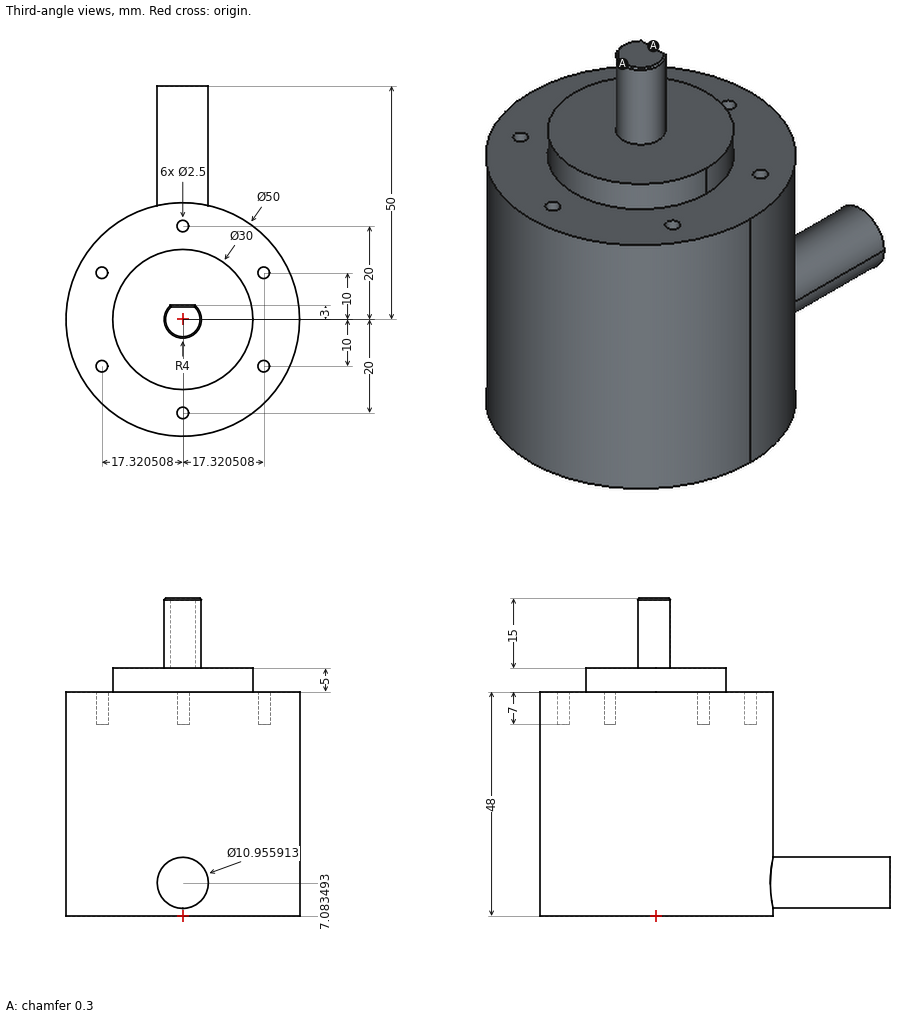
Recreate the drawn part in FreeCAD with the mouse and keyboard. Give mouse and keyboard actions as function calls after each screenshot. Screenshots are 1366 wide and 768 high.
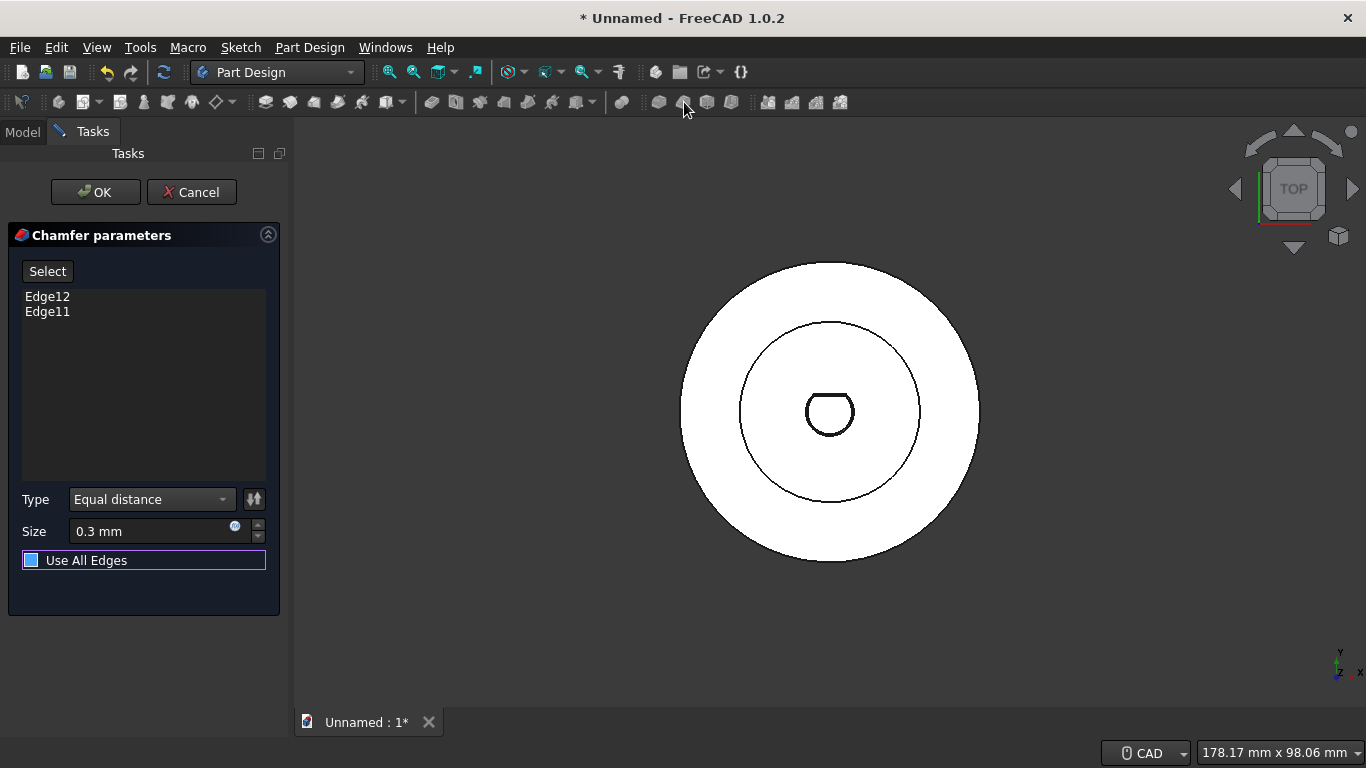
click(96, 192)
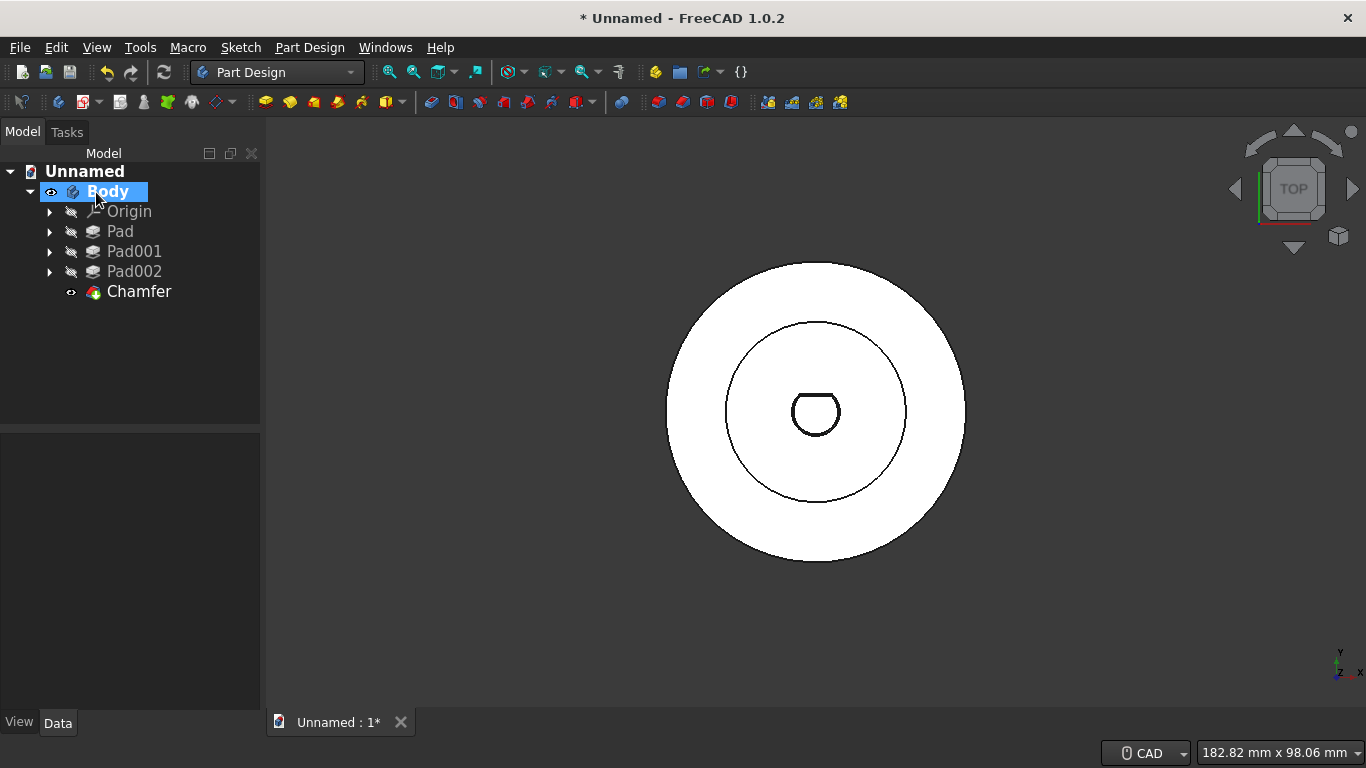
click(84, 102)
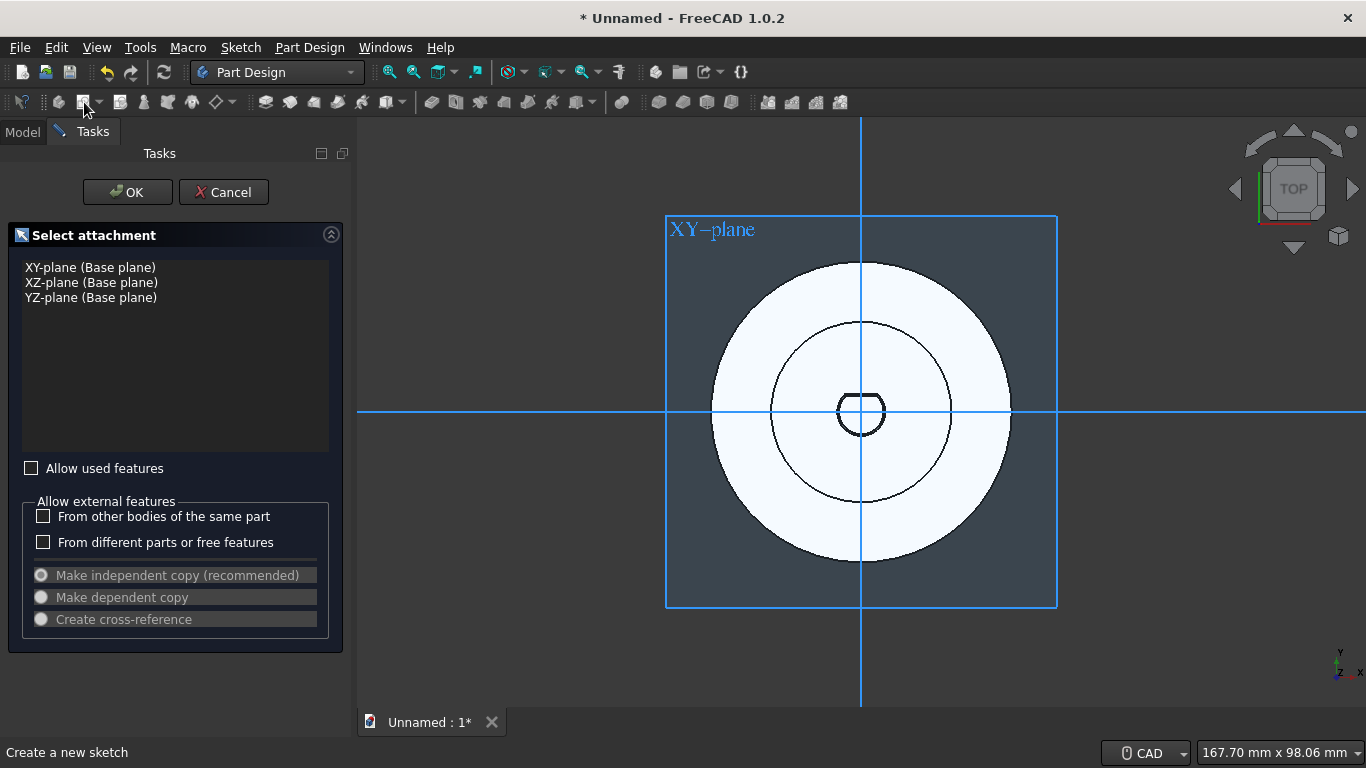
click(82, 282)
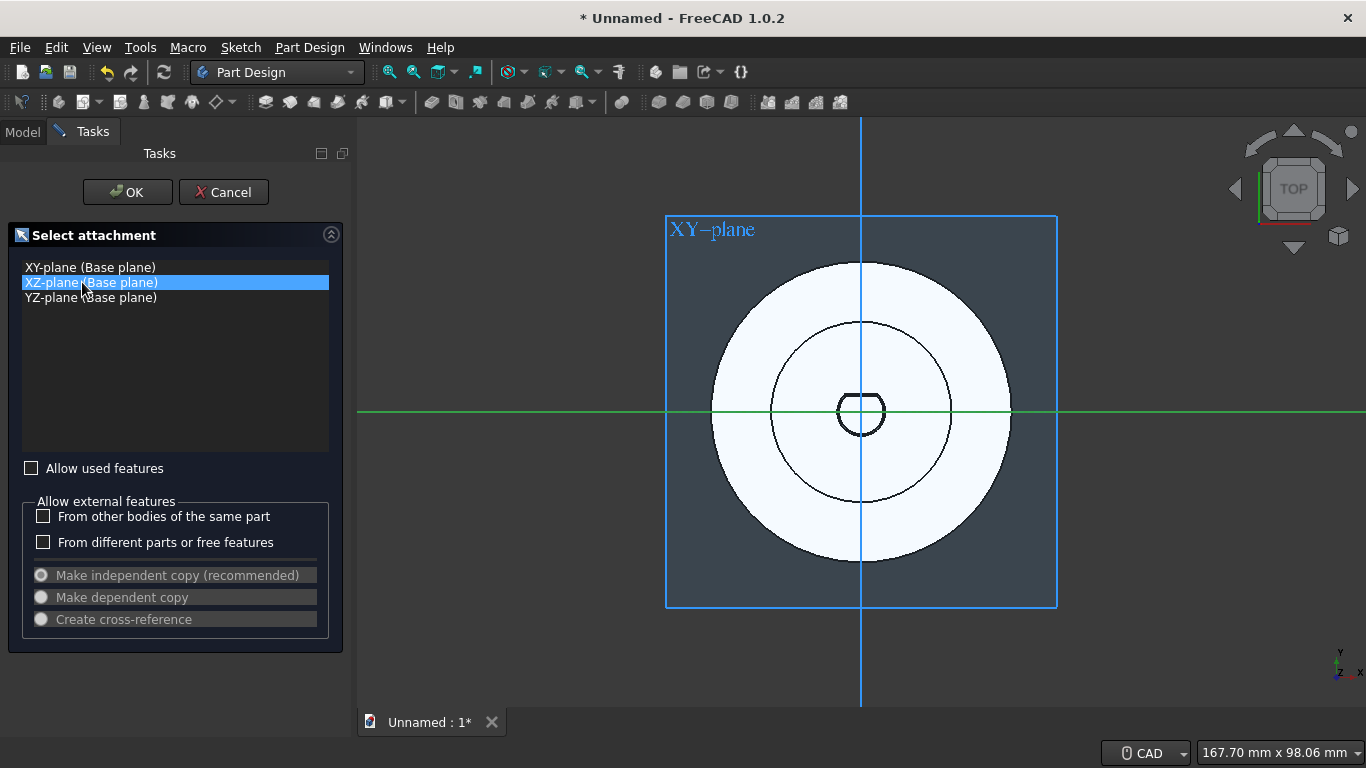
click(128, 192)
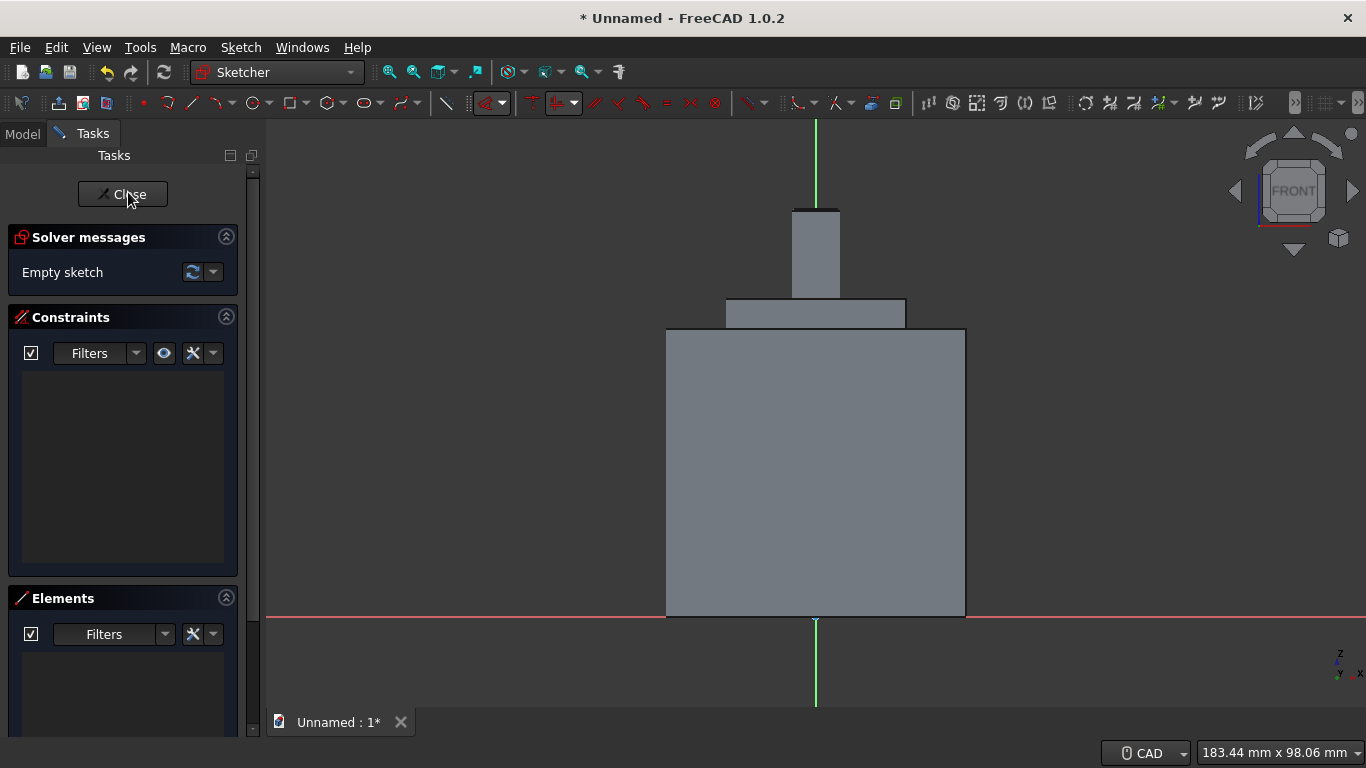
key(q)
key(s)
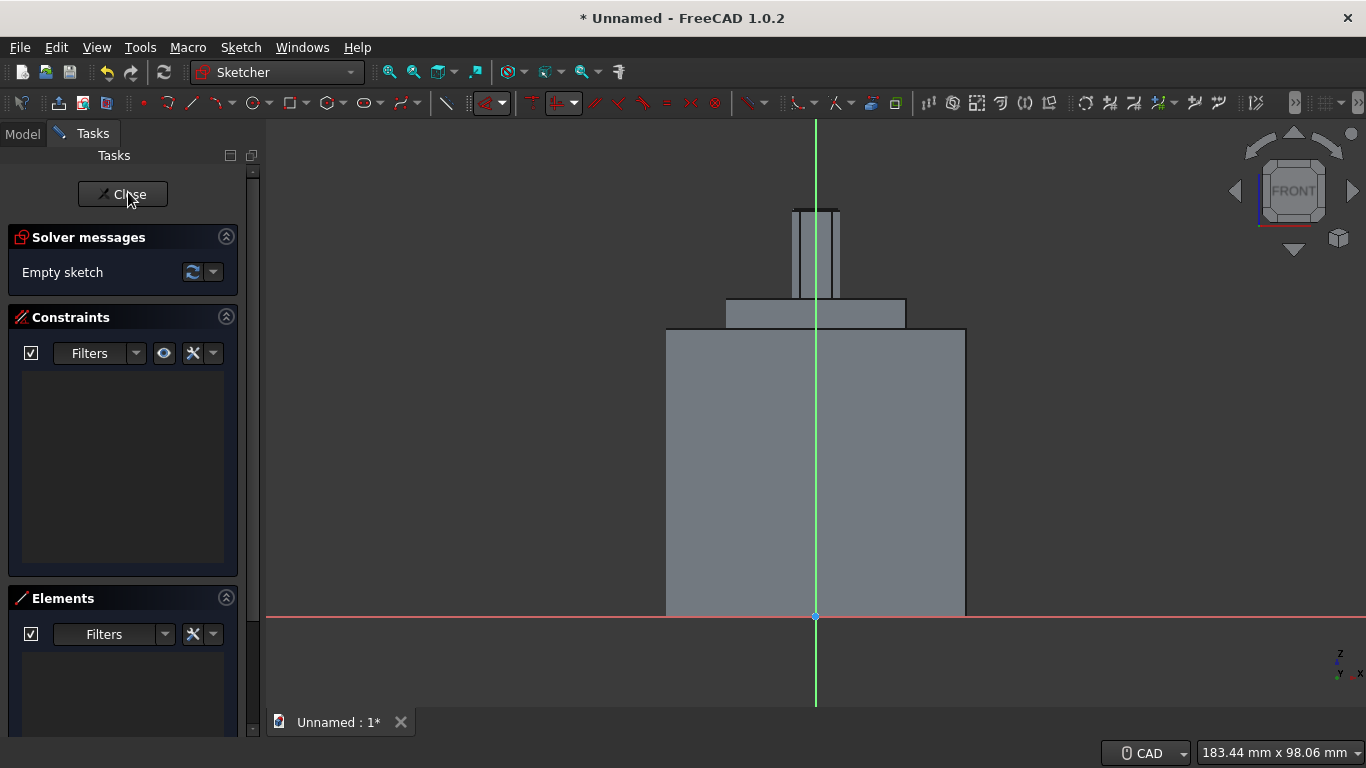
scroll(833, 621, up, 8)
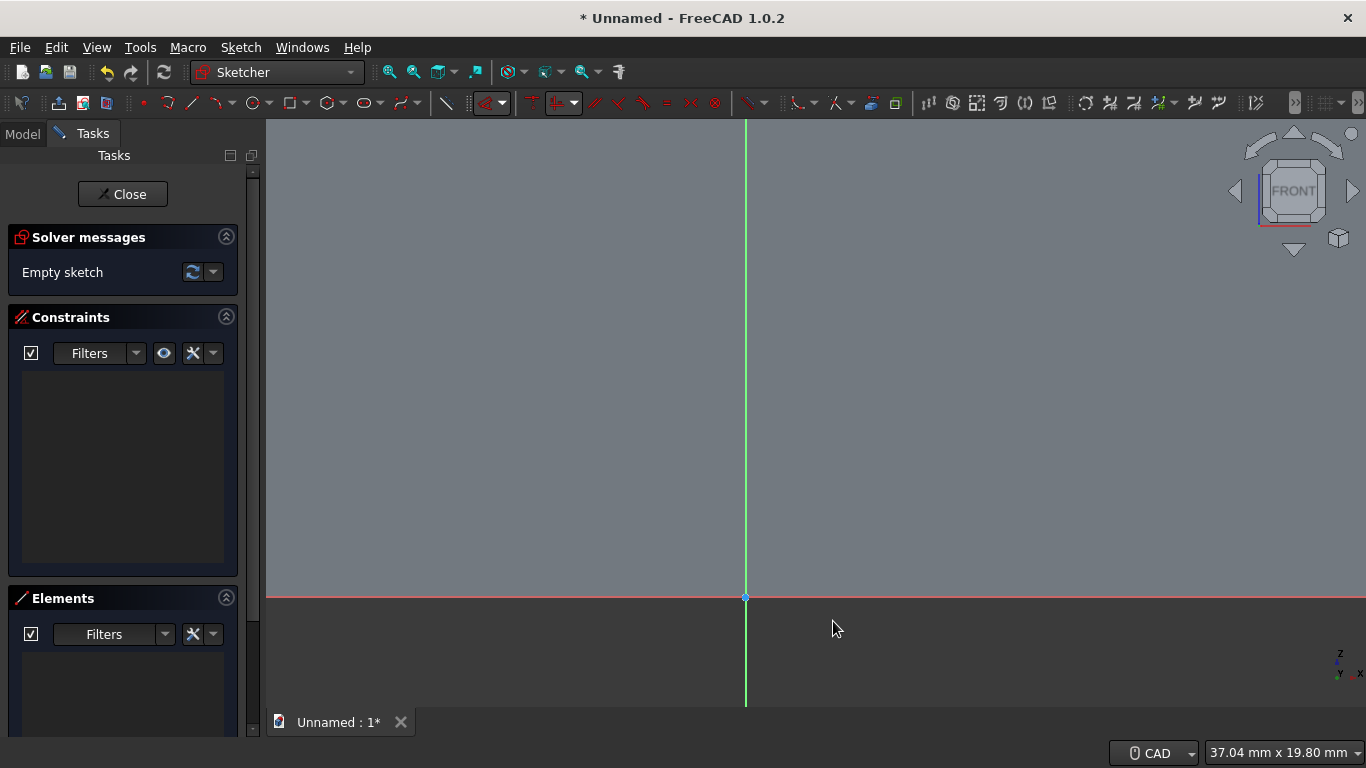
click(254, 104)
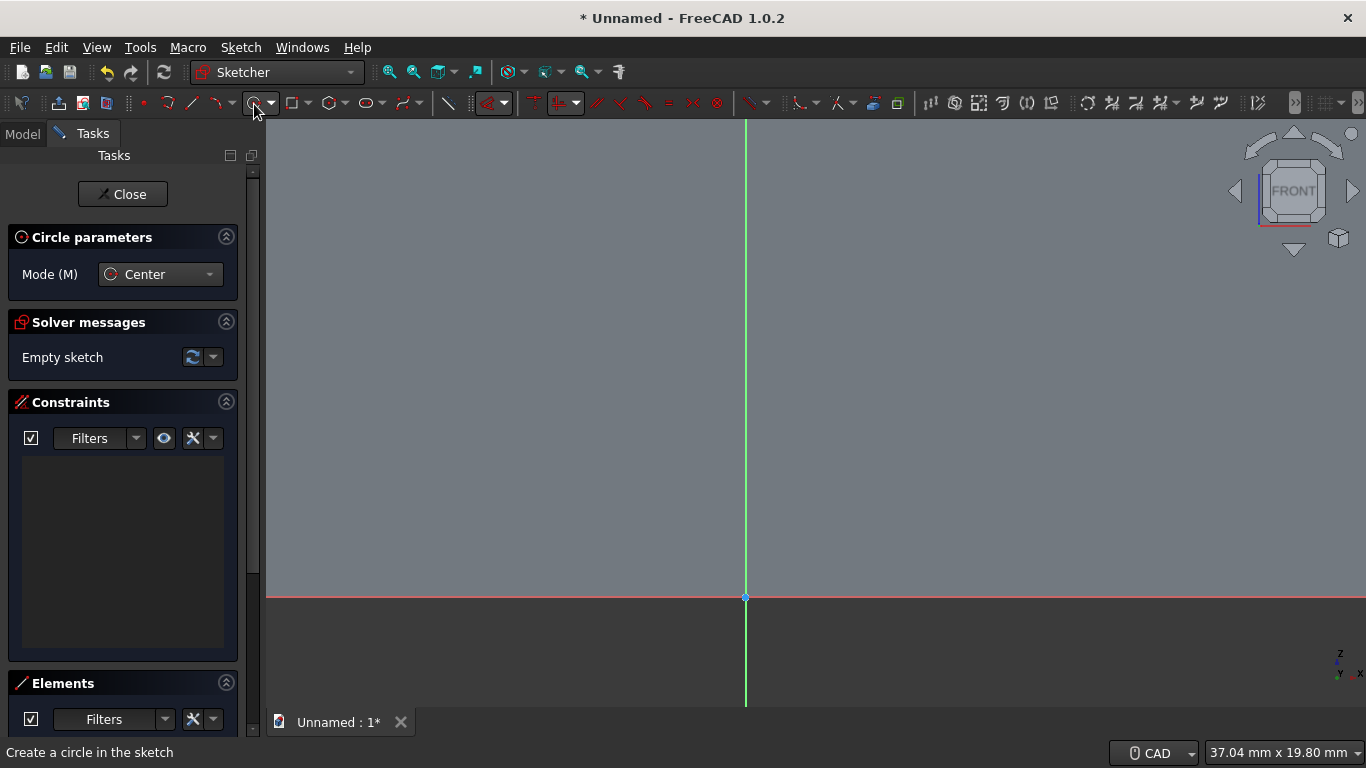
click(746, 387)
move(861, 272)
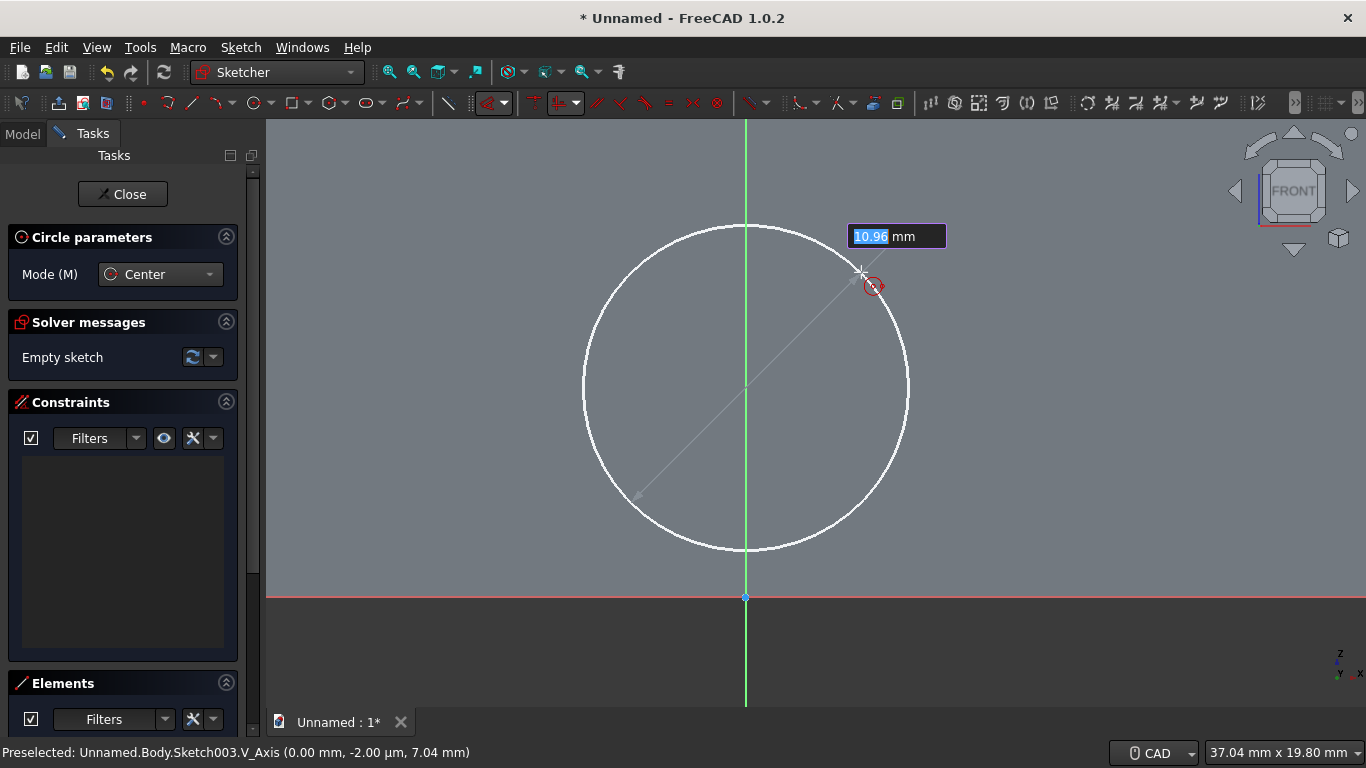
text(10.955913)
key(Return)
key(Escape)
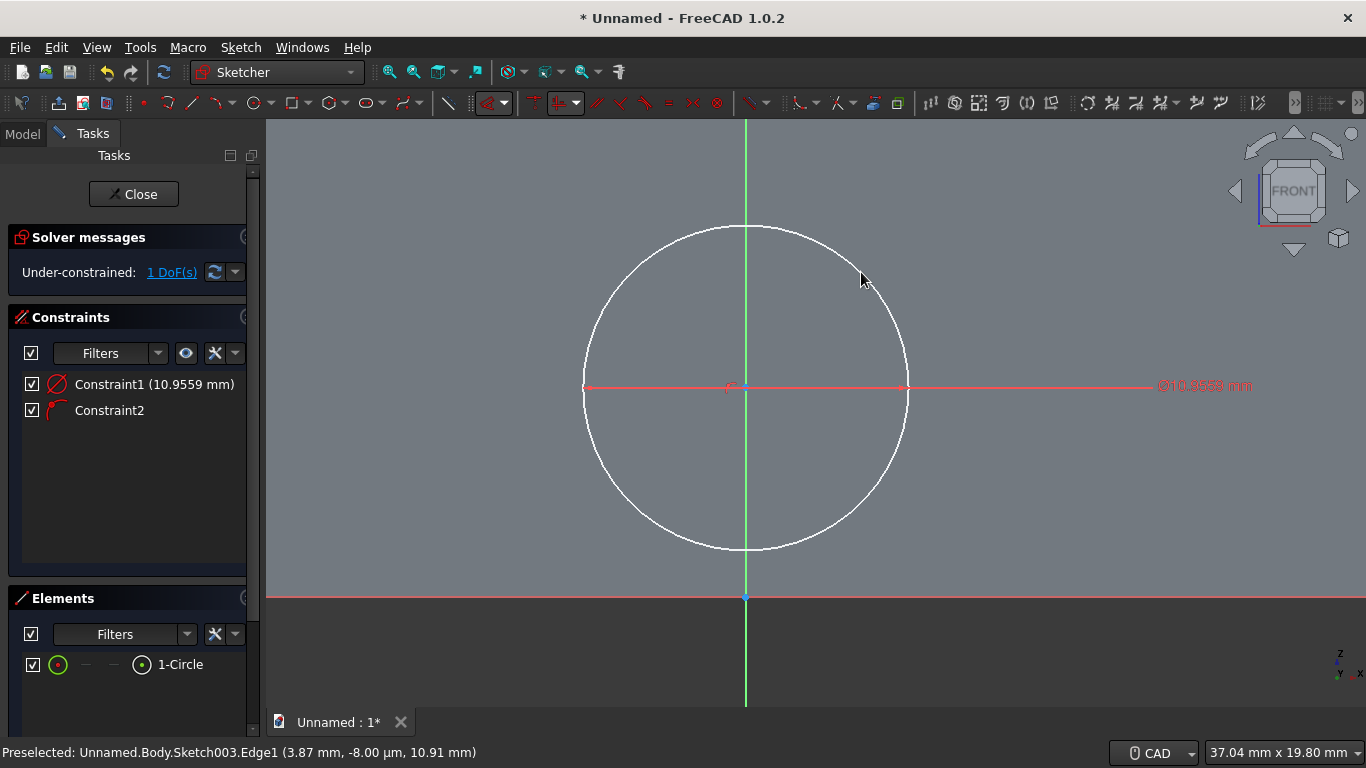
click(746, 388)